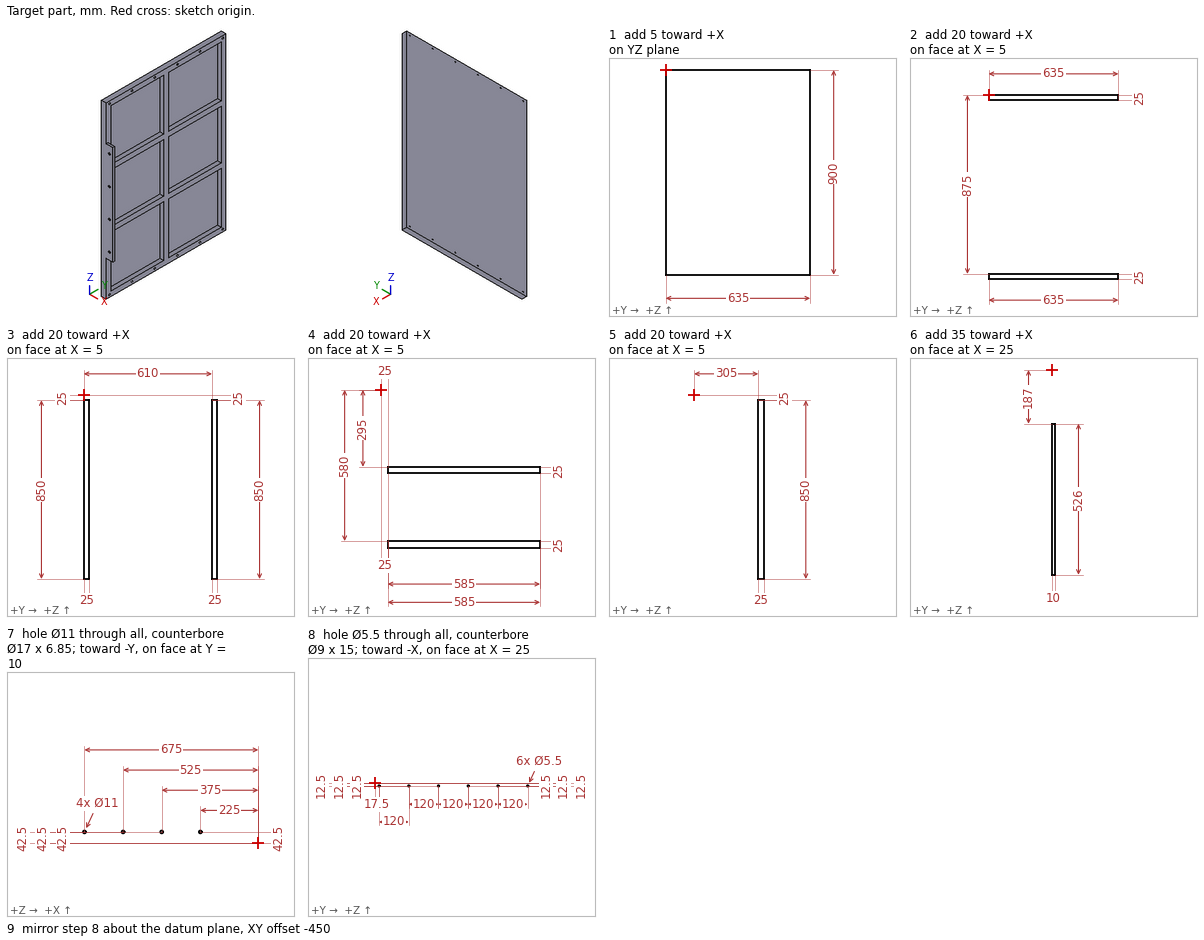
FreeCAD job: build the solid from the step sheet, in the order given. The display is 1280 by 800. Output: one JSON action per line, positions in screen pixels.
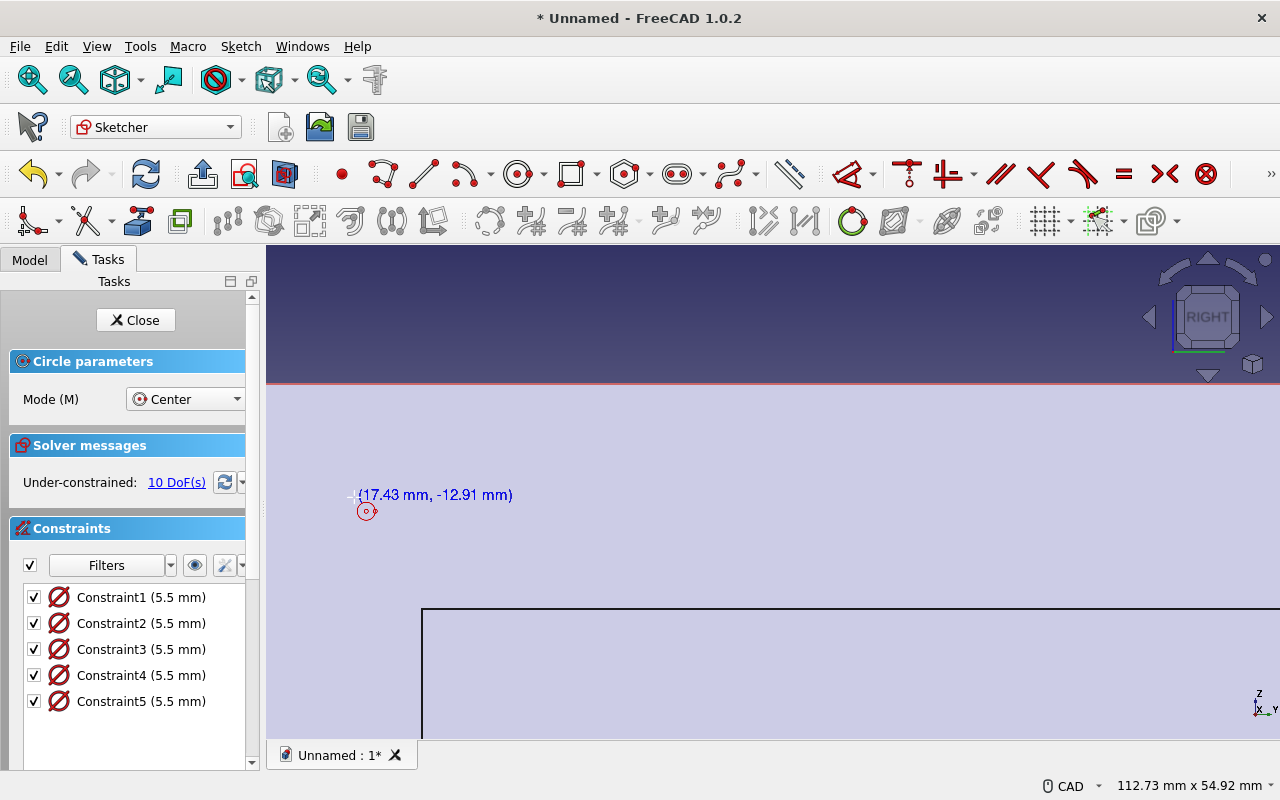
{"action": "scroll", "coordinate": [420, 497], "scroll_direction": "down", "scroll_amount": 11}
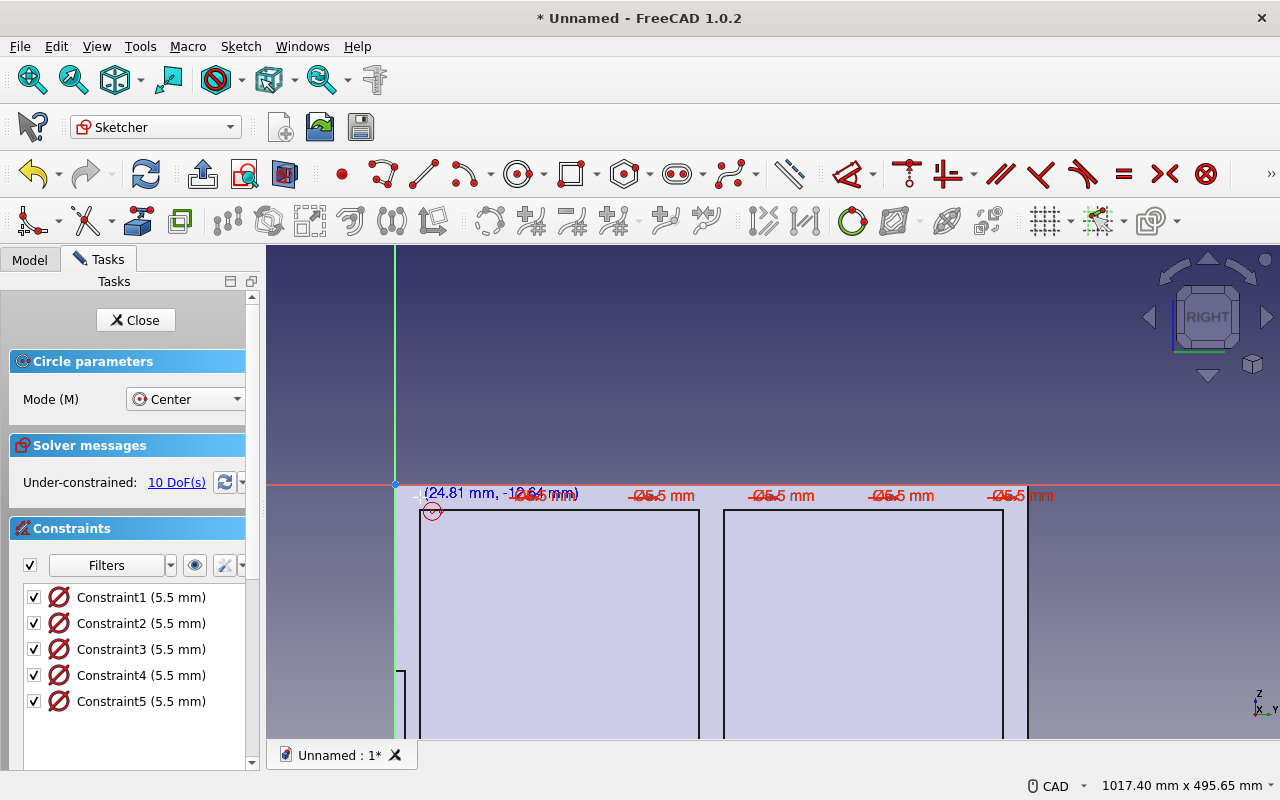
{"action": "scroll", "coordinate": [413, 497], "scroll_direction": "up", "scroll_amount": 2}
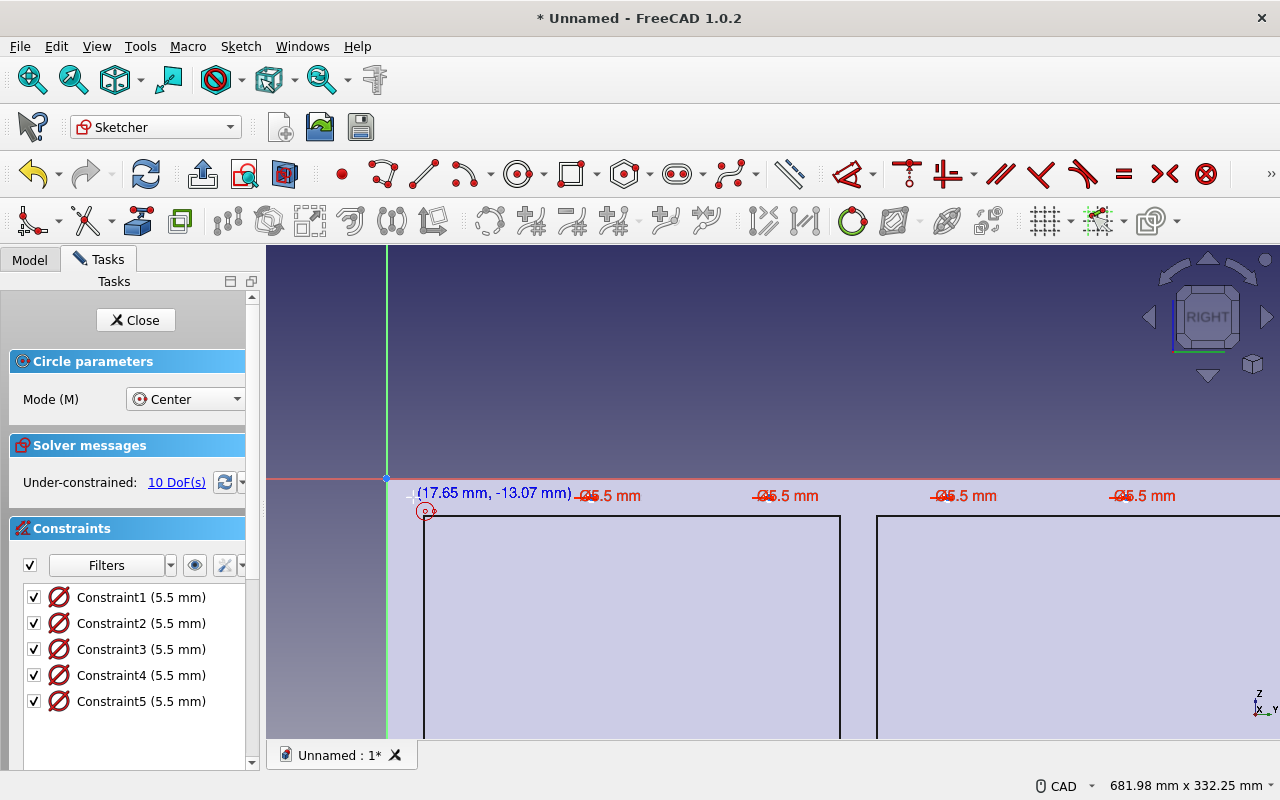
{"action": "left_click", "coordinate": [413, 497]}
{"action": "mouse_move", "coordinate": [416, 494]}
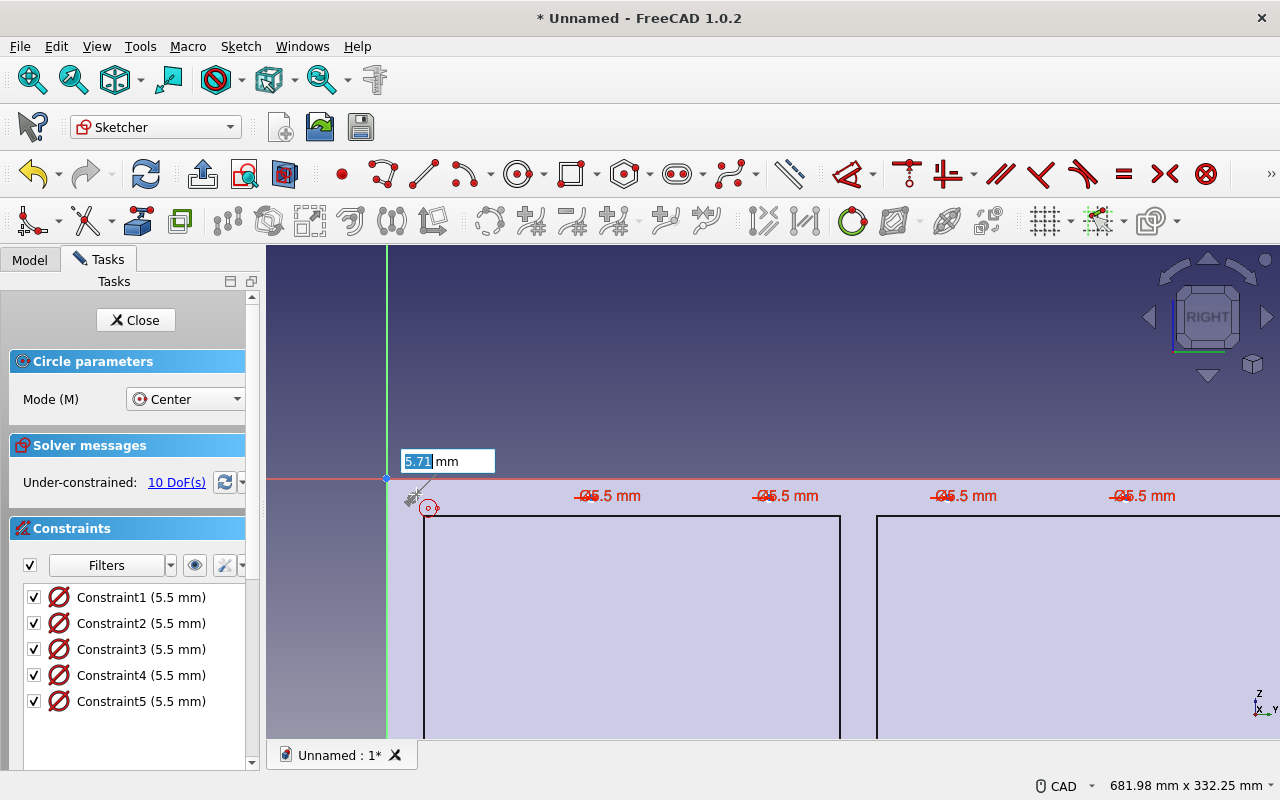
{"action": "type", "text": "5.5"}
{"action": "key", "text": "Return"}
{"action": "key", "text": "Escape"}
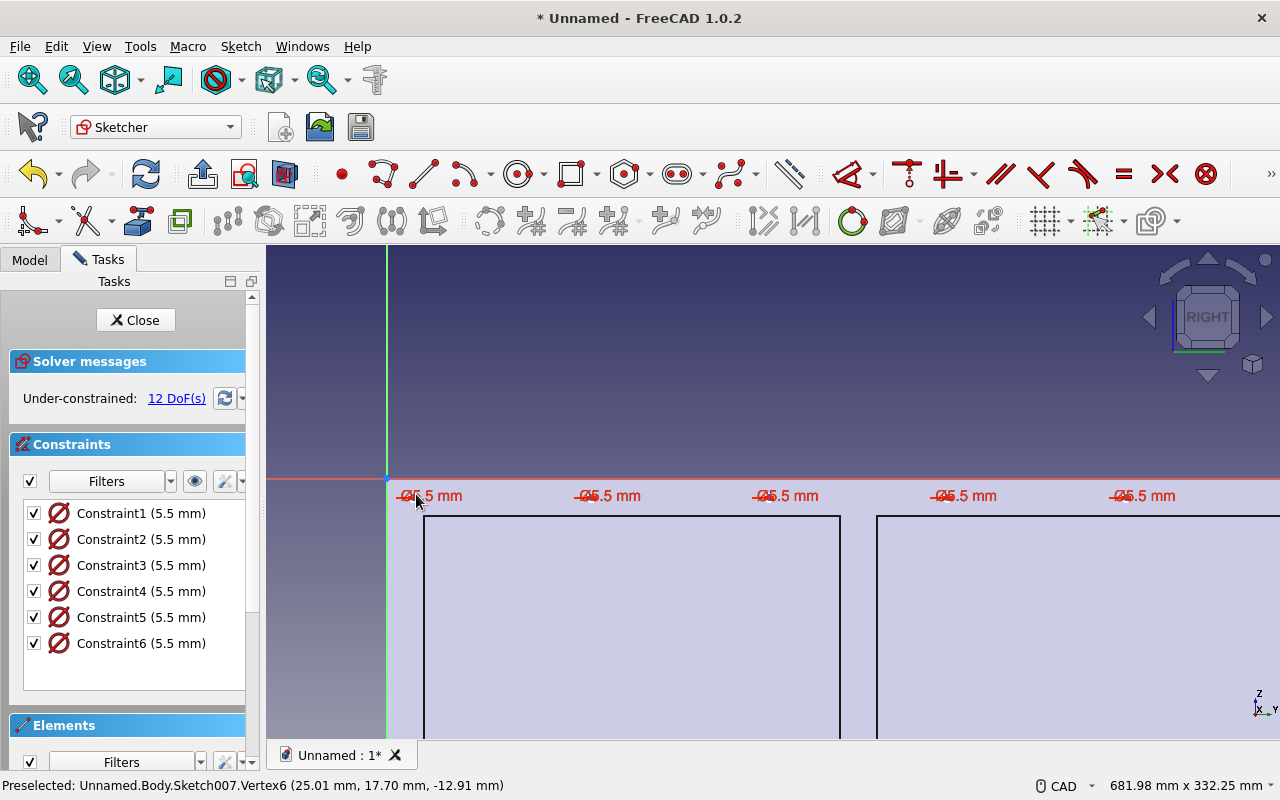
{"action": "left_click", "coordinate": [846, 174]}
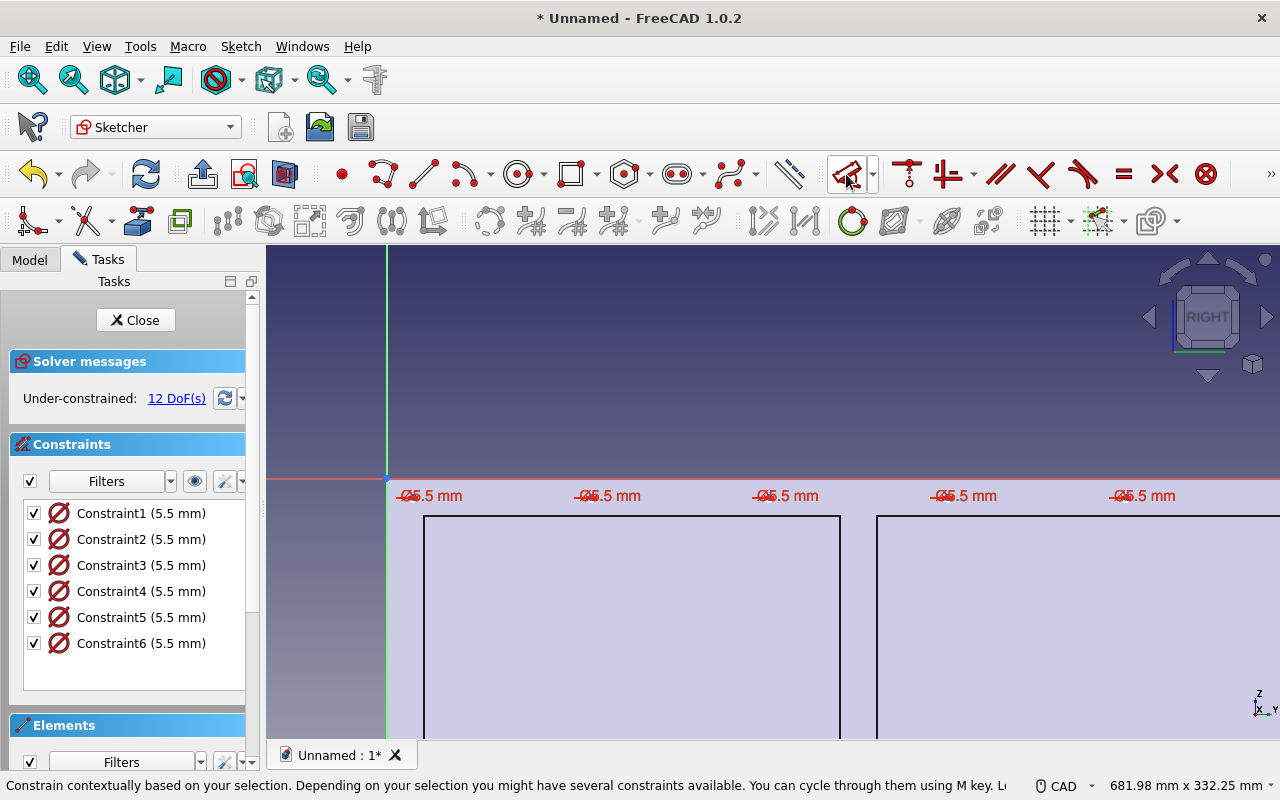
{"action": "scroll", "coordinate": [413, 496], "scroll_direction": "down", "scroll_amount": 2}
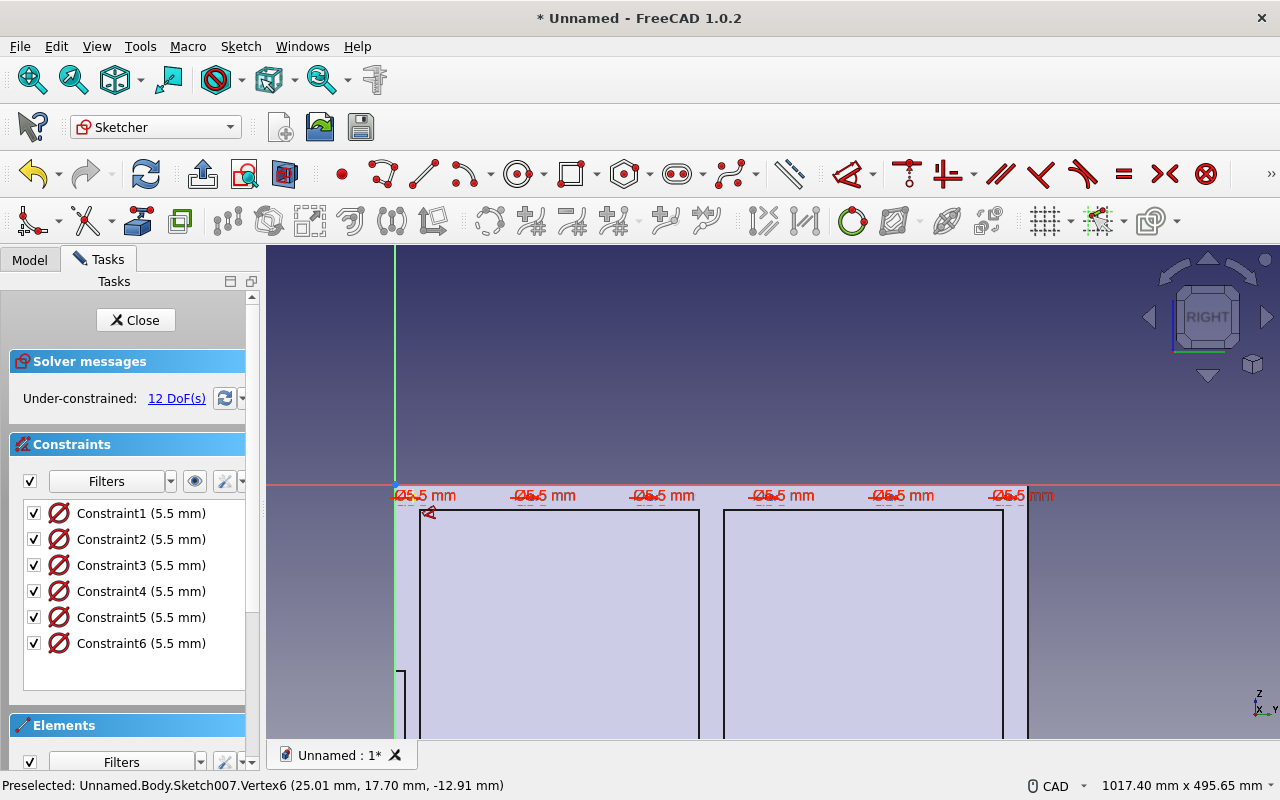
{"action": "scroll", "coordinate": [1011, 498], "scroll_direction": "up", "scroll_amount": 6}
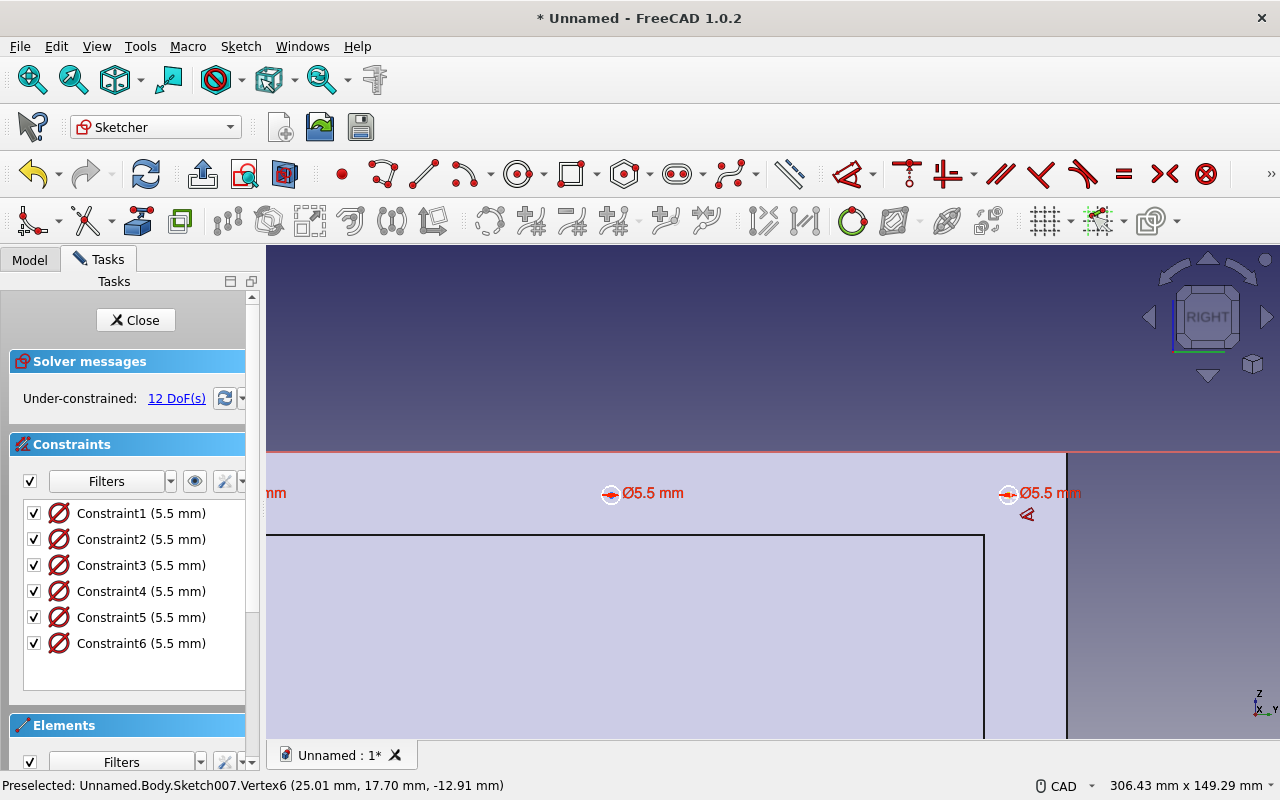
{"action": "left_click", "coordinate": [1009, 495]}
{"action": "left_click", "coordinate": [1043, 474]}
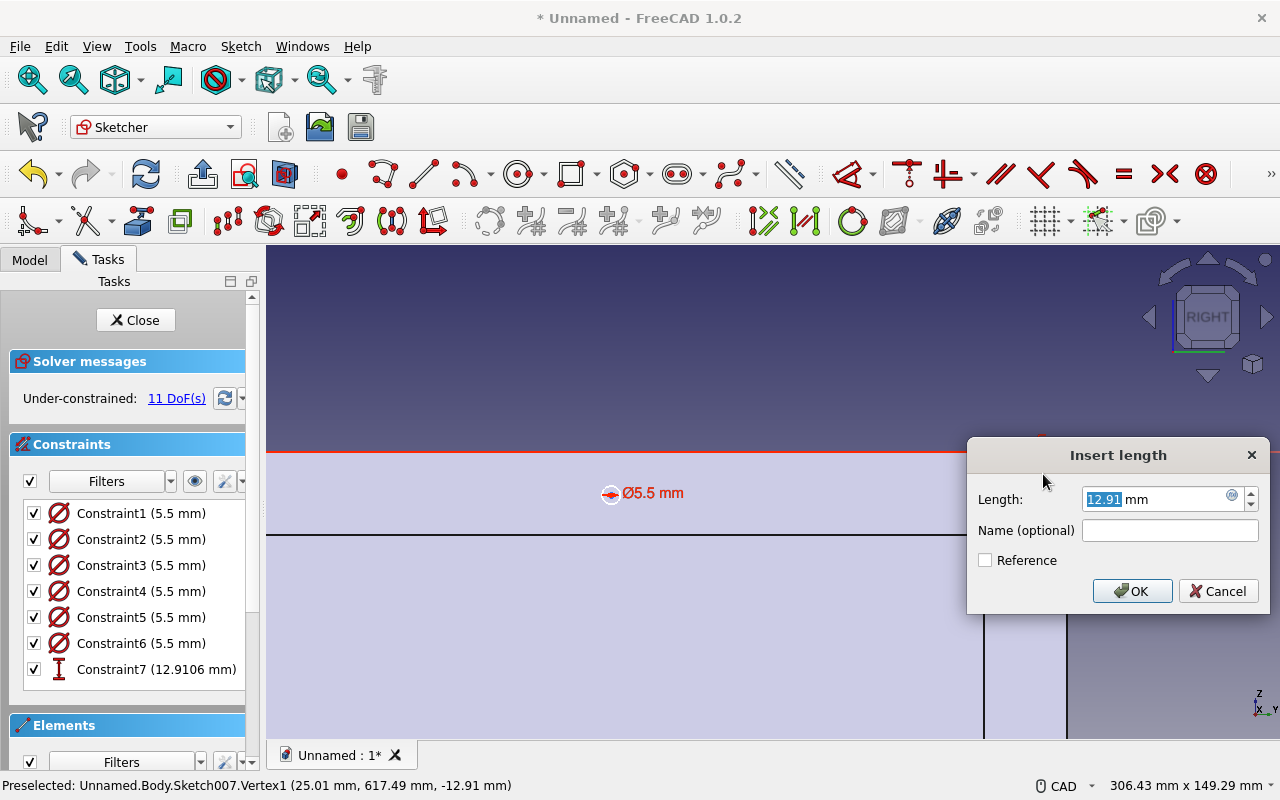
{"action": "type", "text": "12.5"}
{"action": "key", "text": "Return"}